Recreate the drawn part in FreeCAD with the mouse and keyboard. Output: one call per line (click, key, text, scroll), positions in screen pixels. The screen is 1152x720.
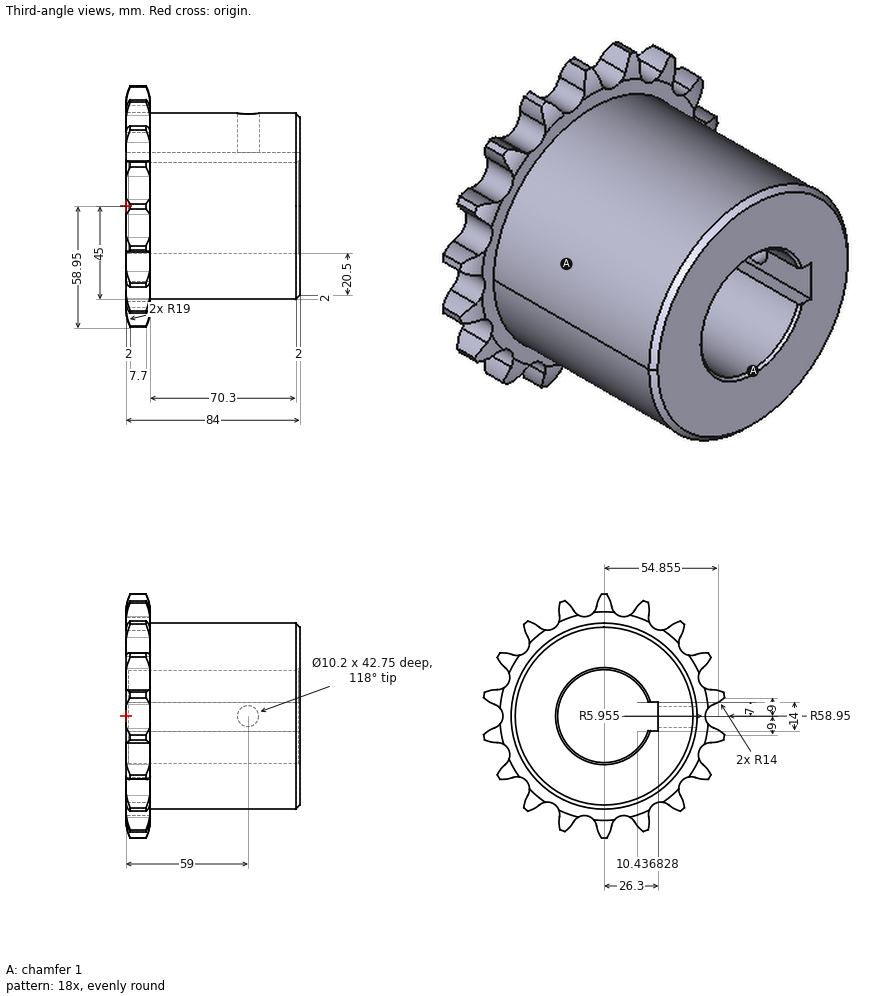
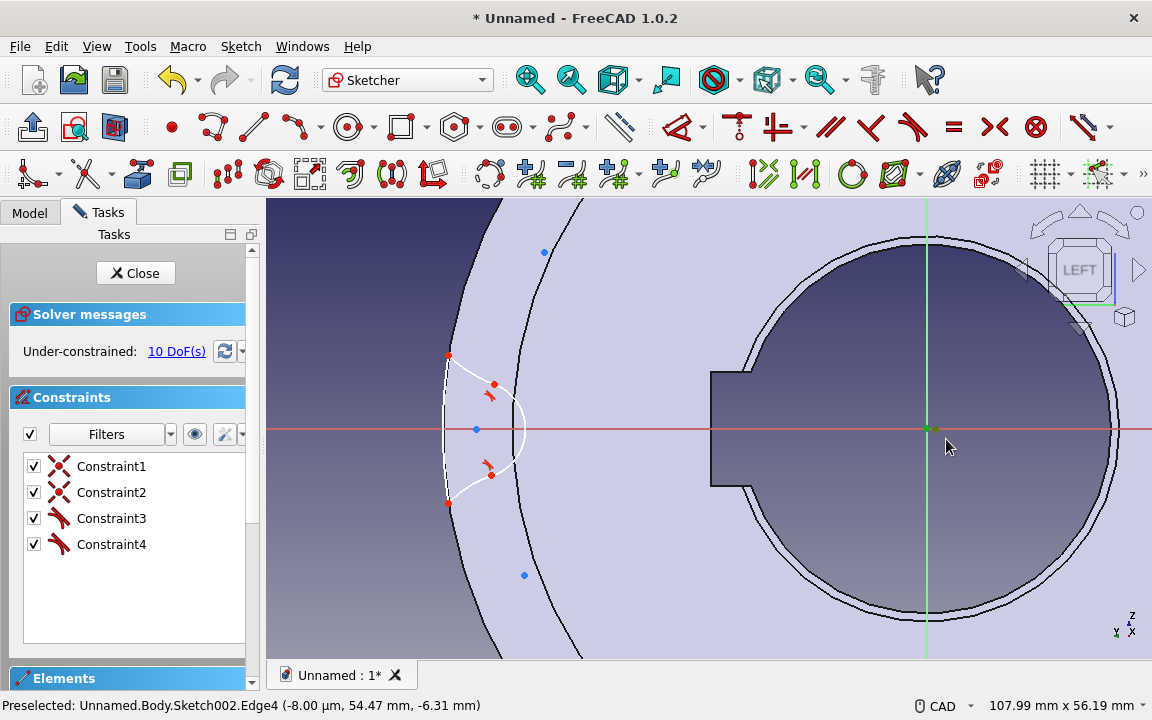
key(c)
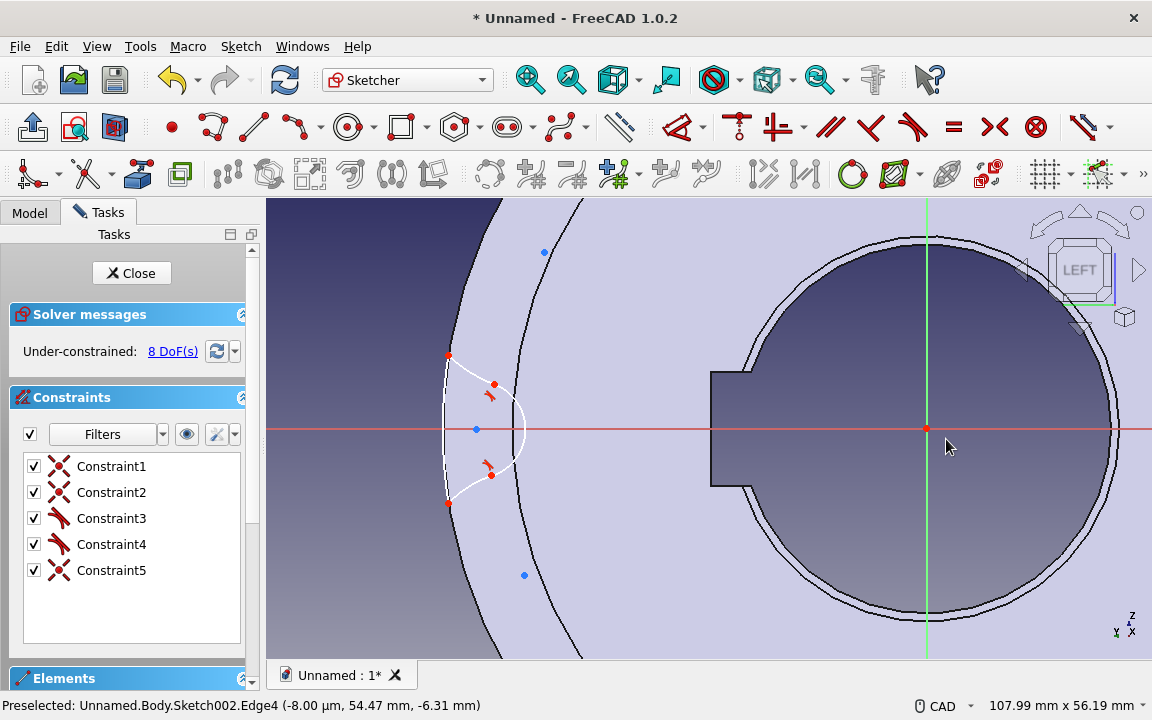
click(461, 366)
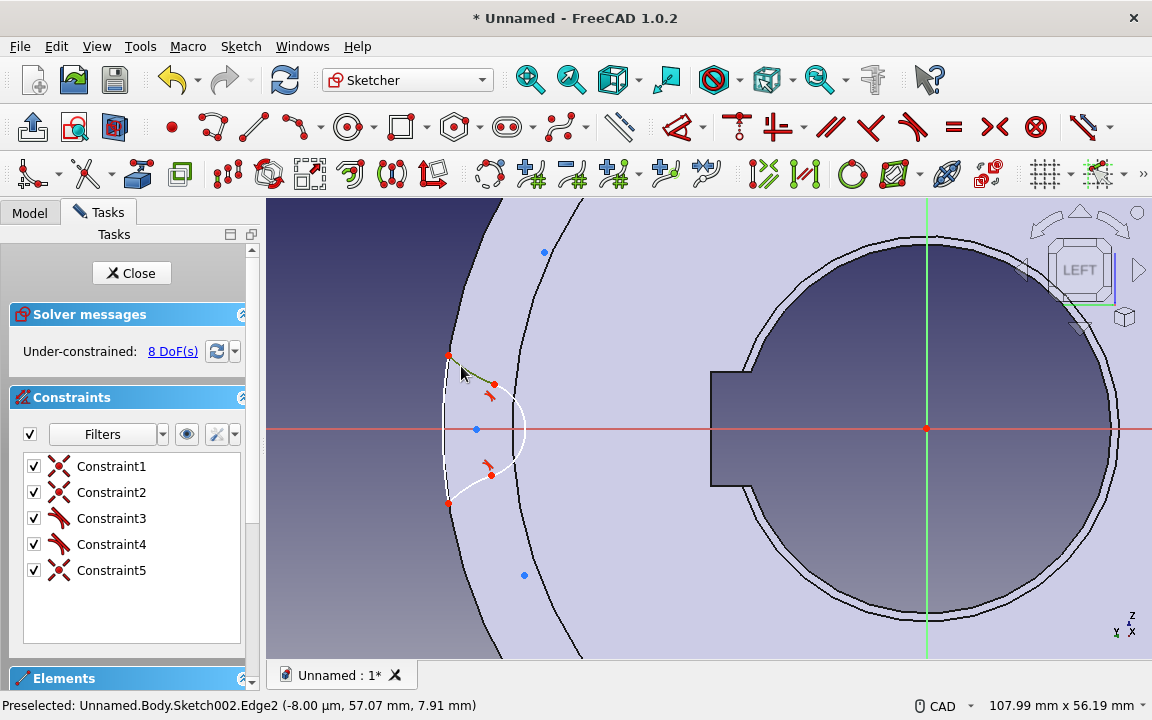
click(478, 482)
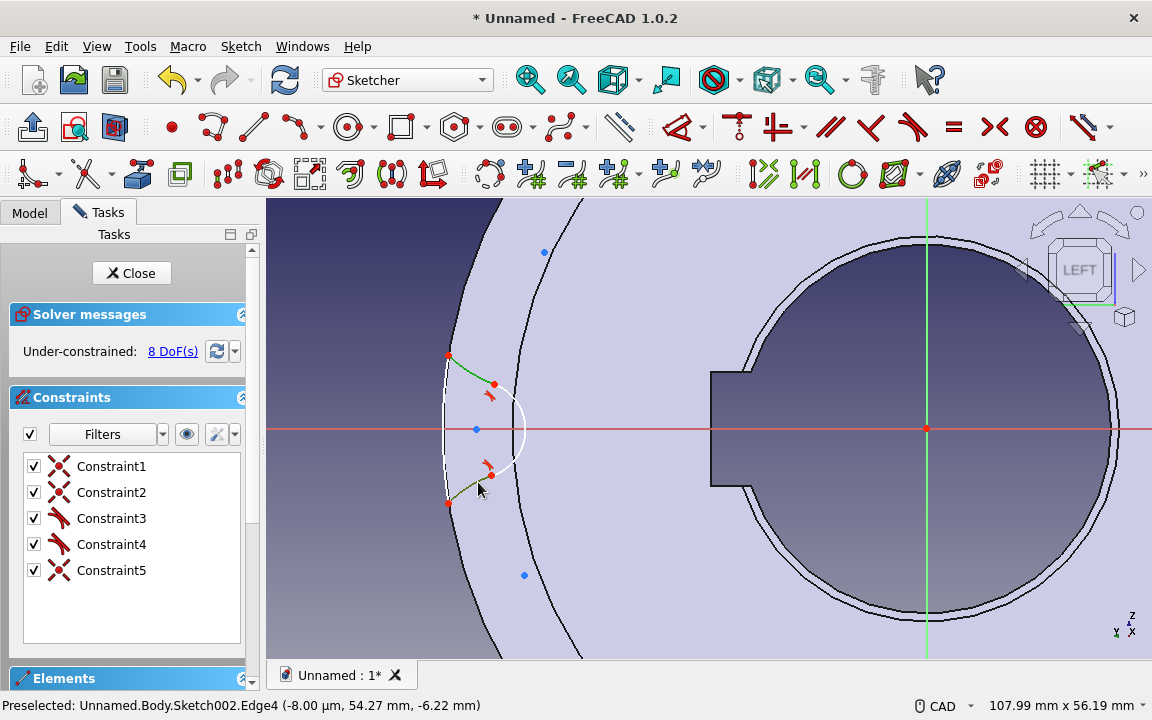
click(954, 128)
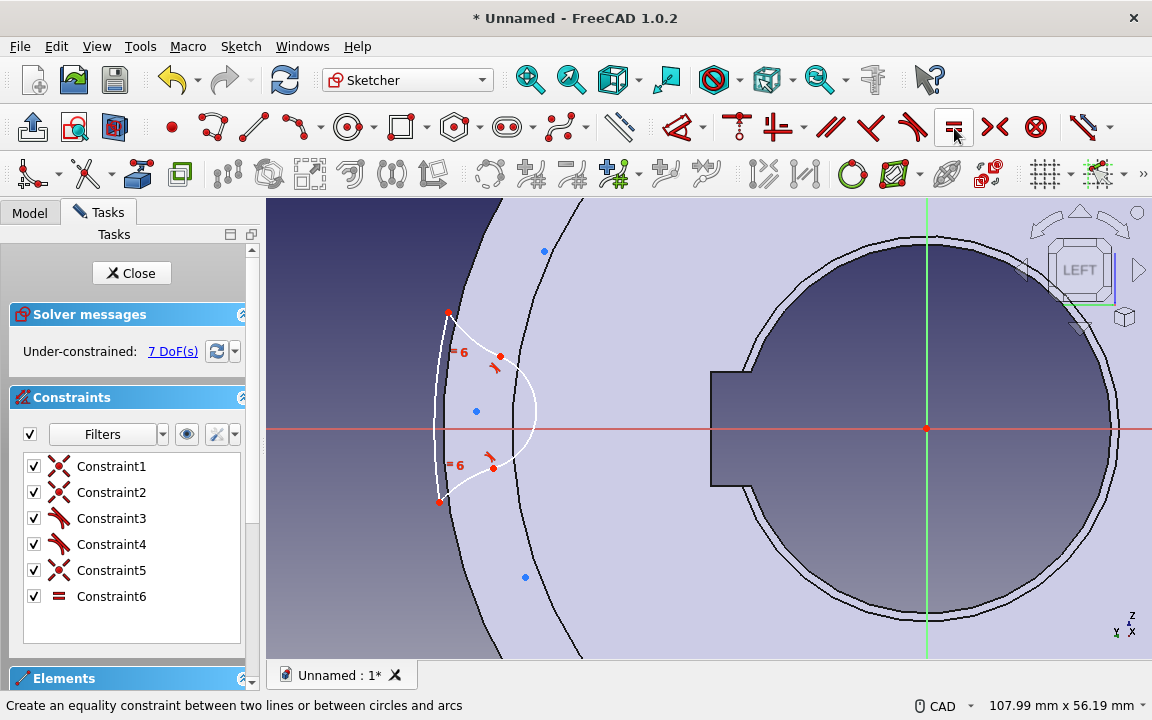
click(477, 411)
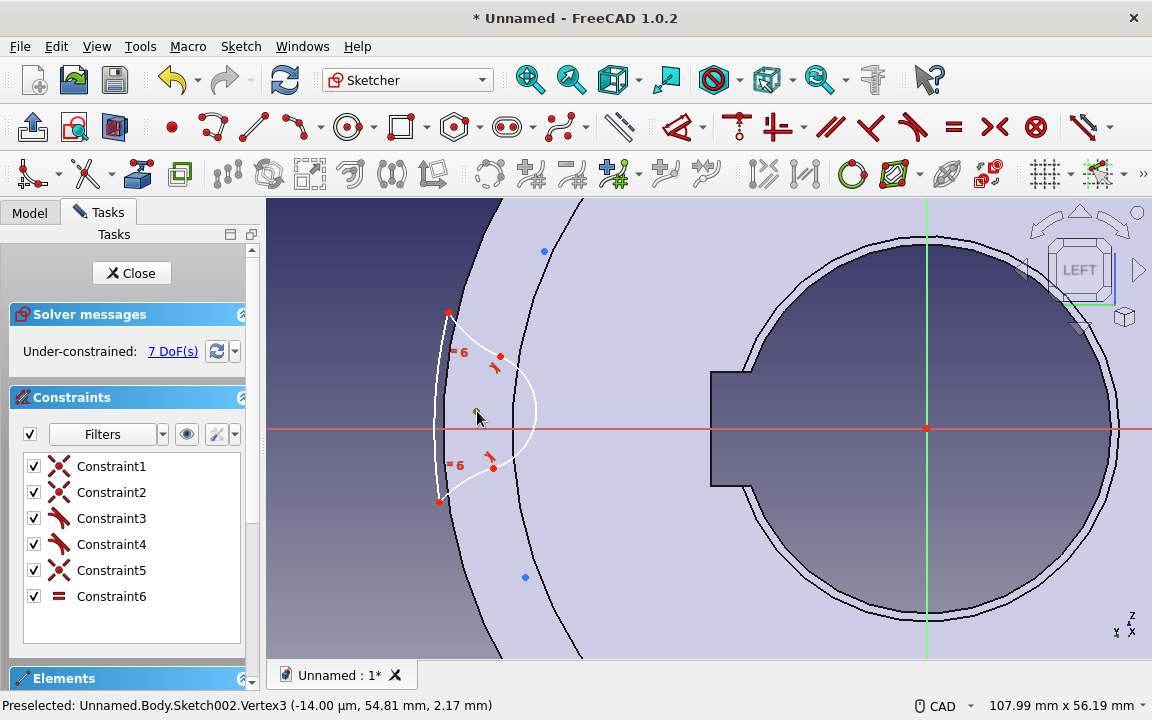
click(344, 429)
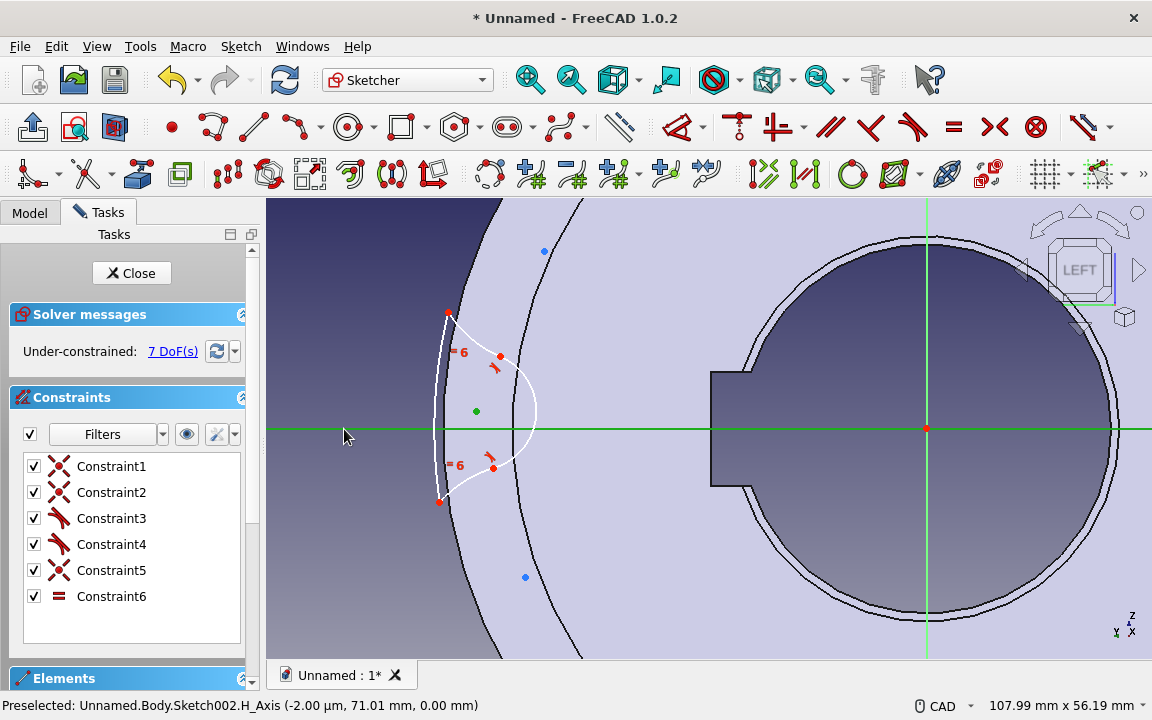
click(737, 128)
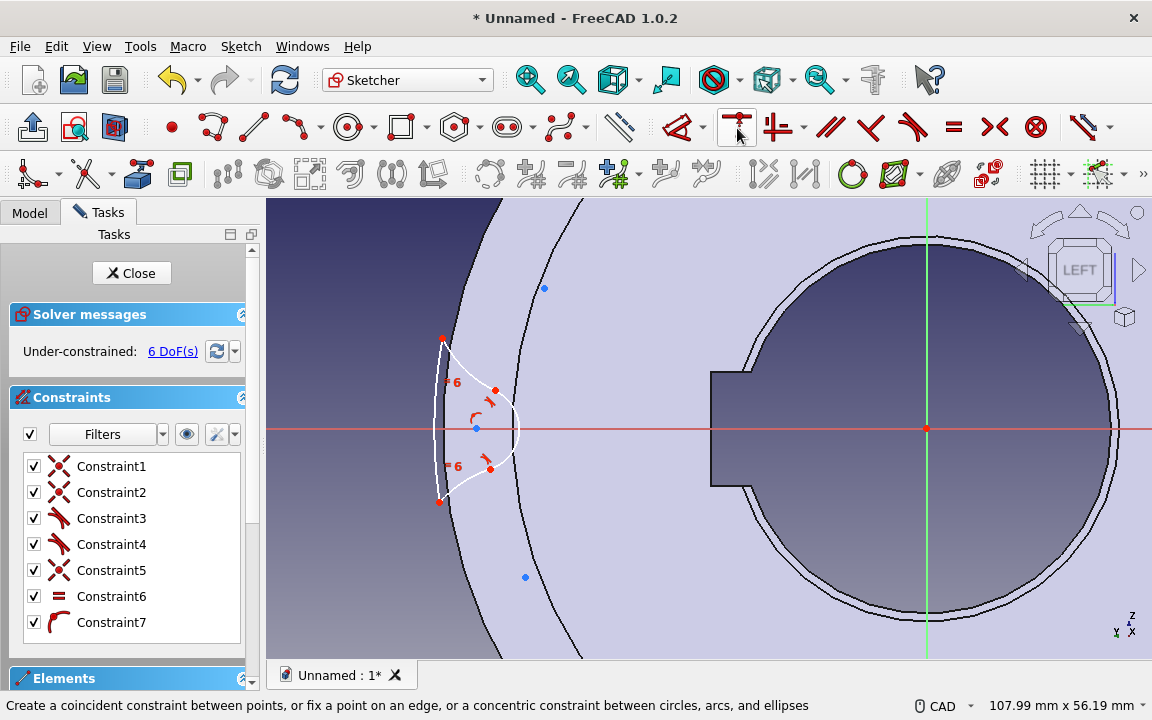
click(676, 128)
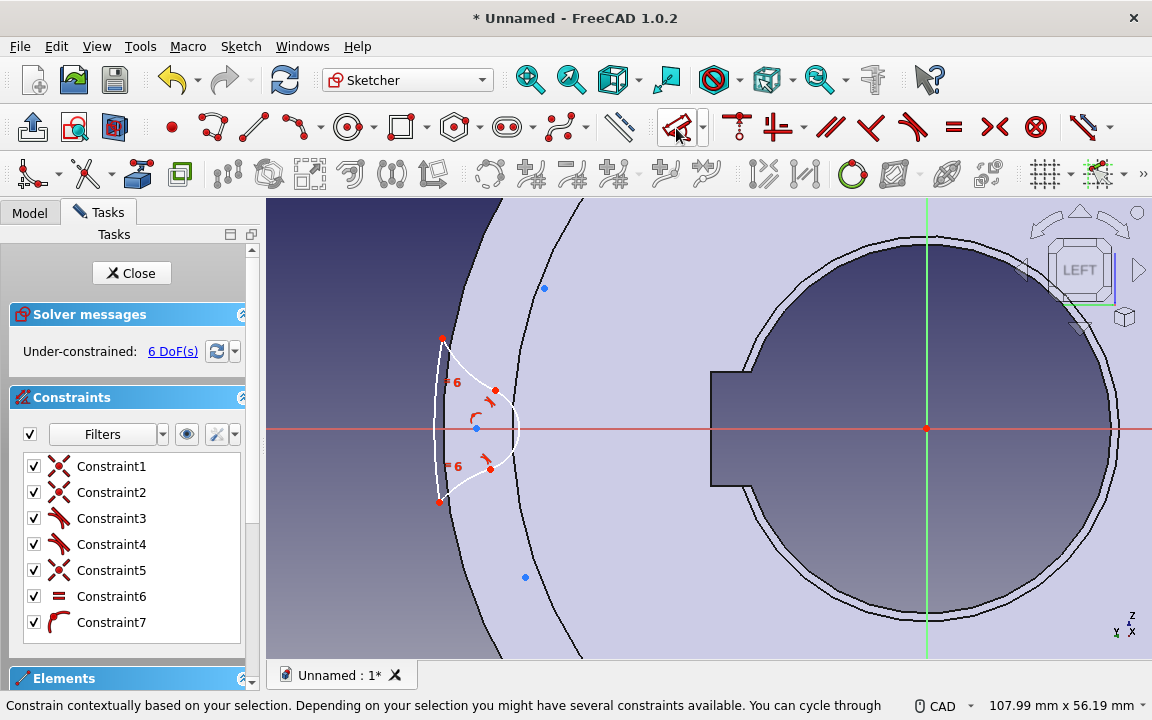
click(513, 451)
click(540, 468)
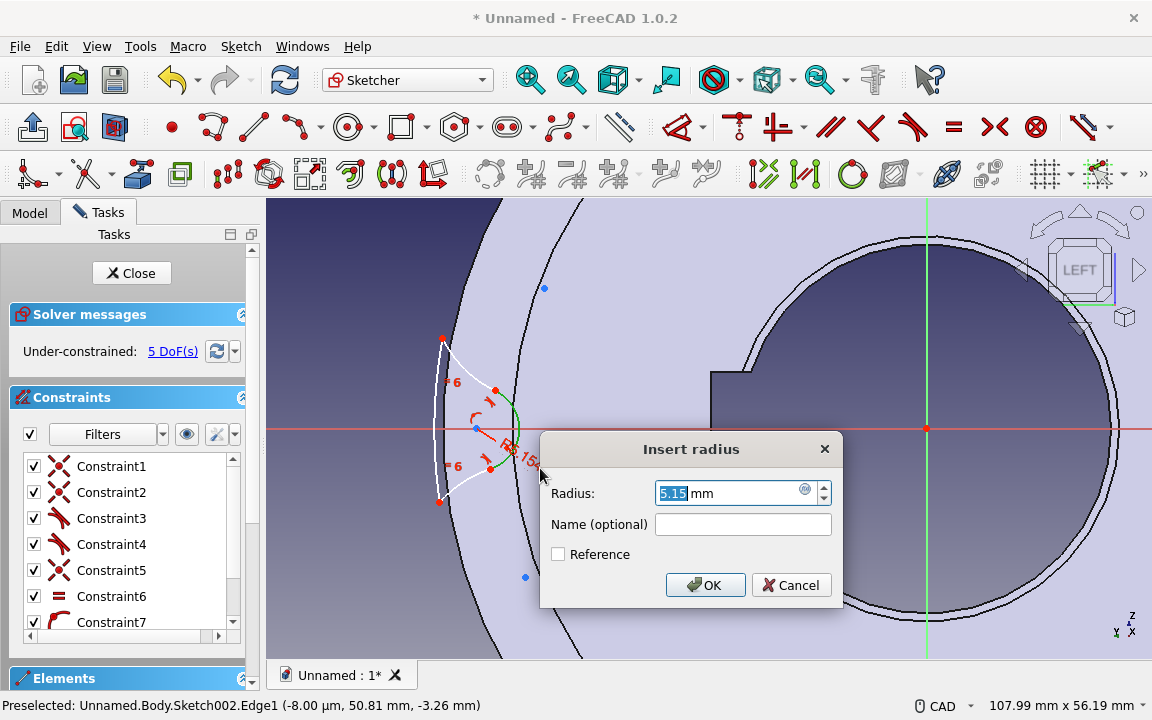
text(5.955)
key(Return)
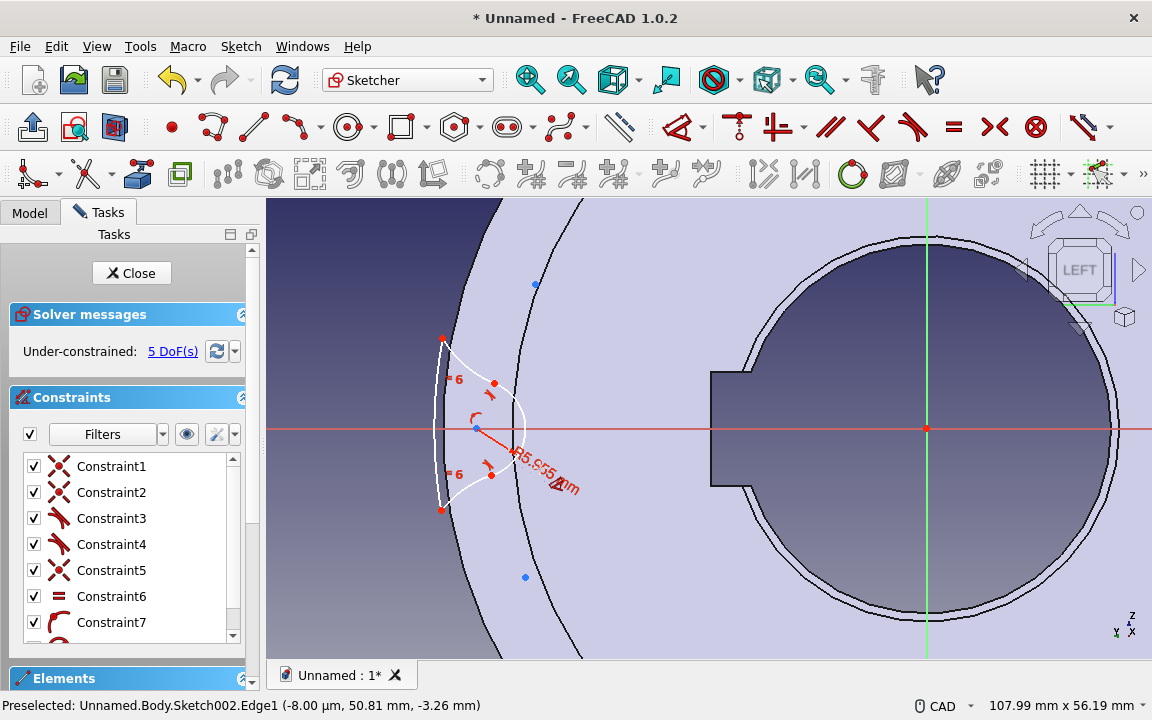
click(455, 356)
click(399, 316)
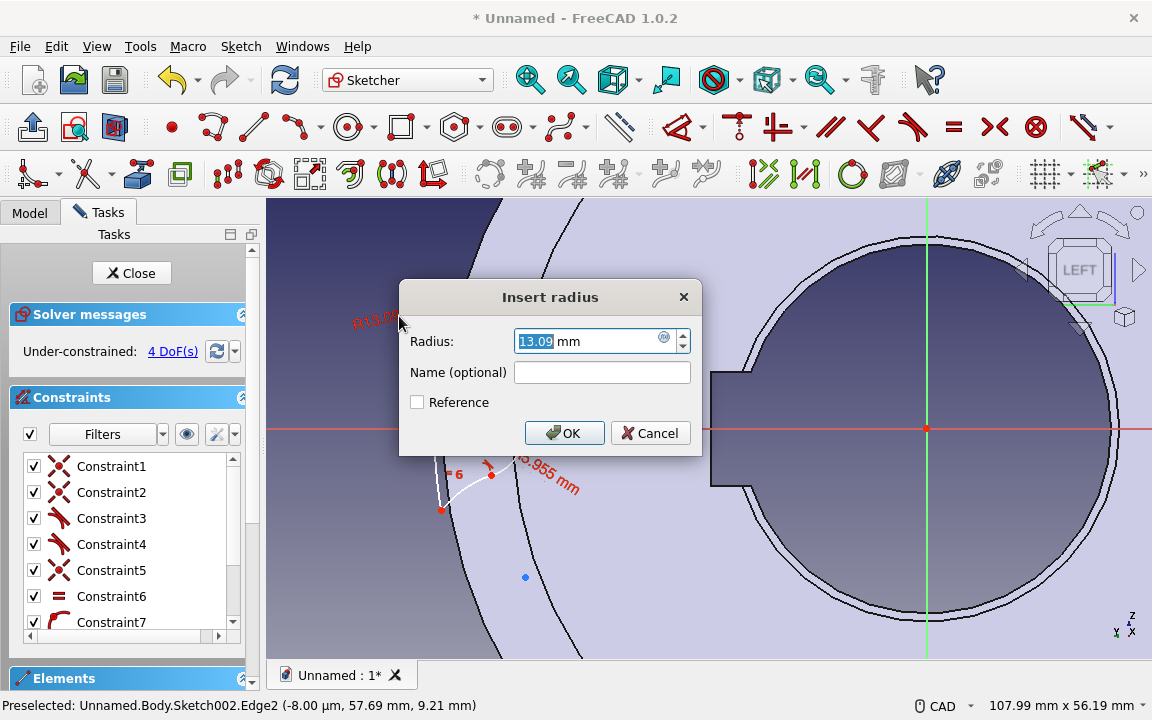
text(14)
key(Return)